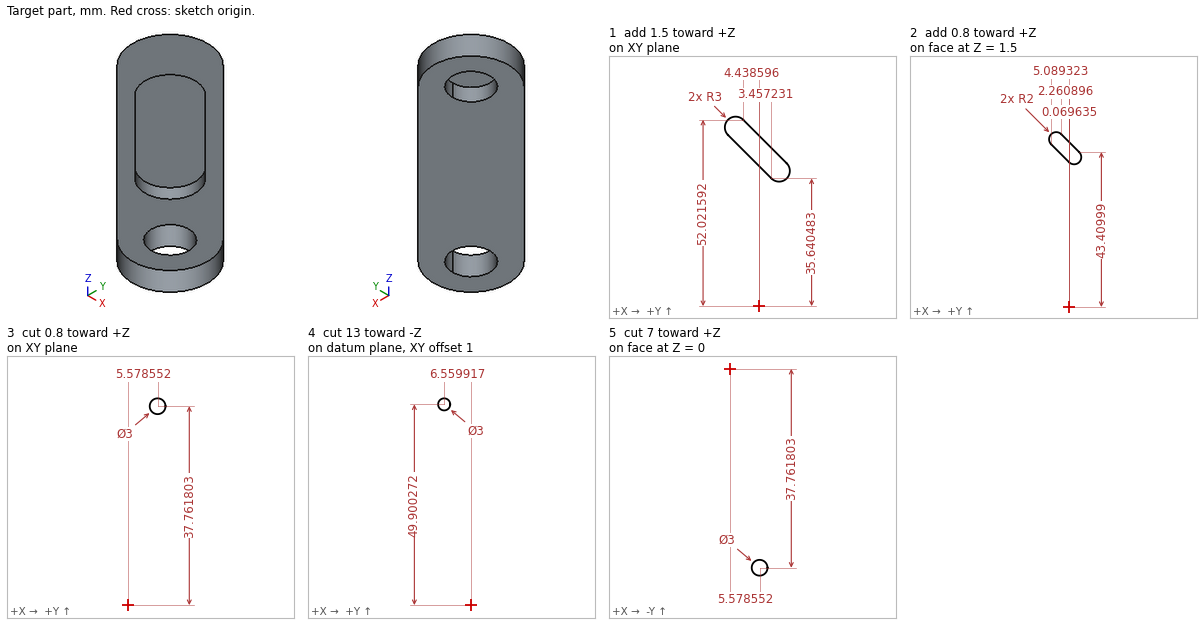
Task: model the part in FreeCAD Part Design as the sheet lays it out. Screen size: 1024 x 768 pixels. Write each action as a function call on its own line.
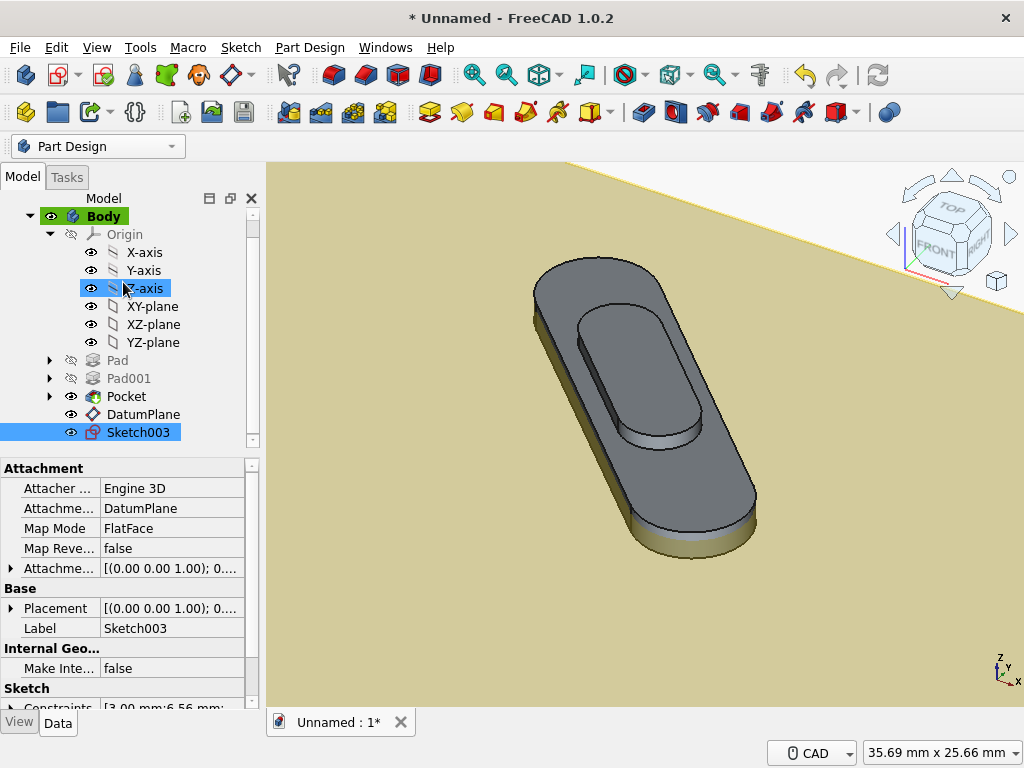
click(644, 112)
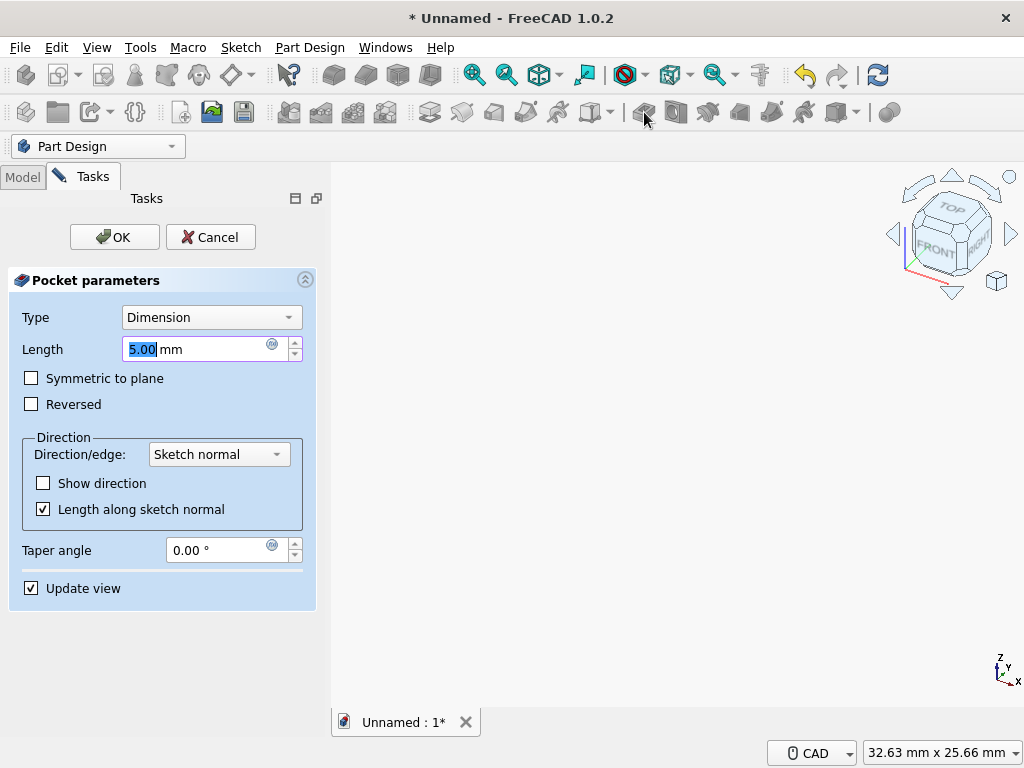
text(13)
key(Tab)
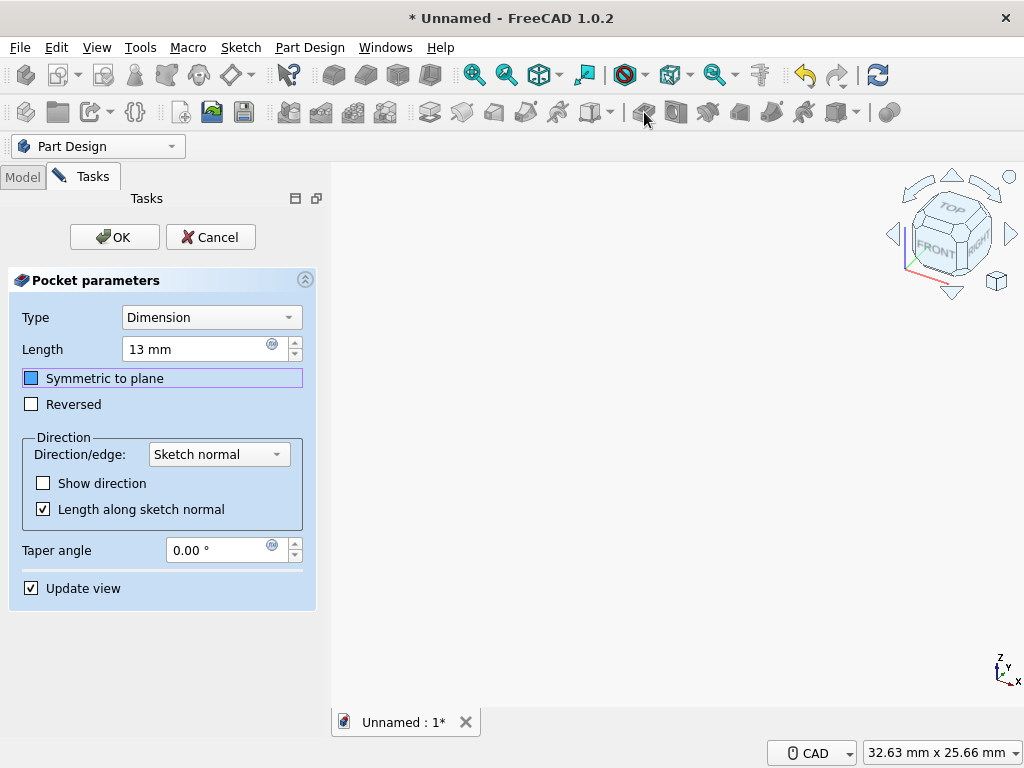
click(115, 237)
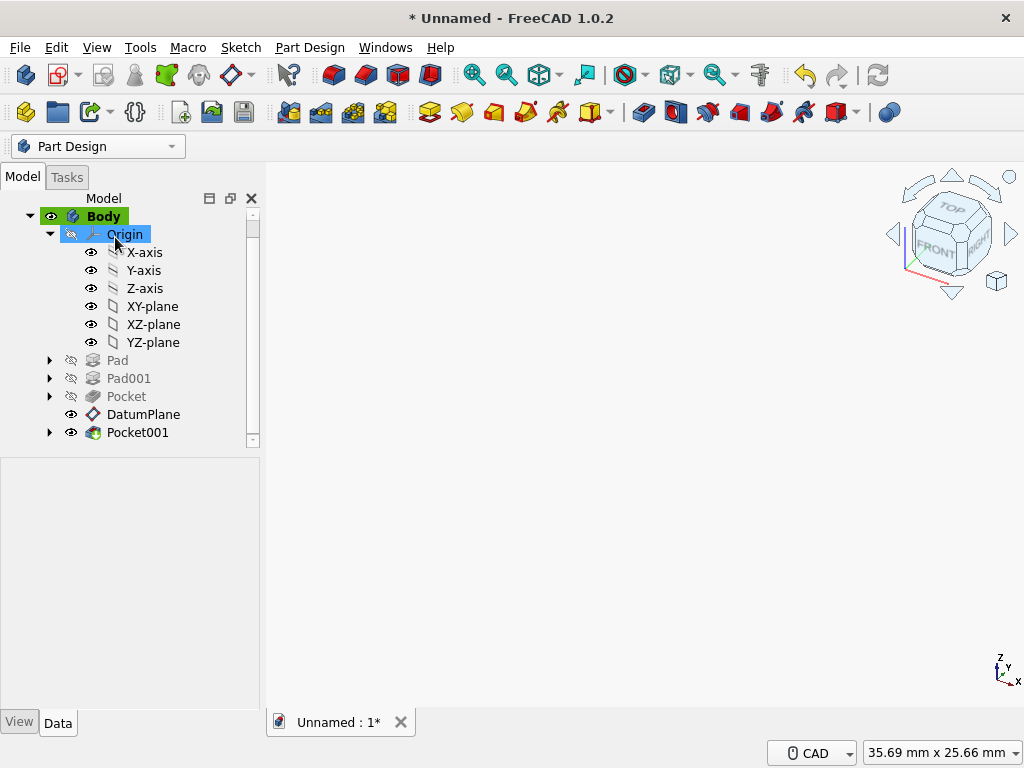
click(116, 414)
key(space)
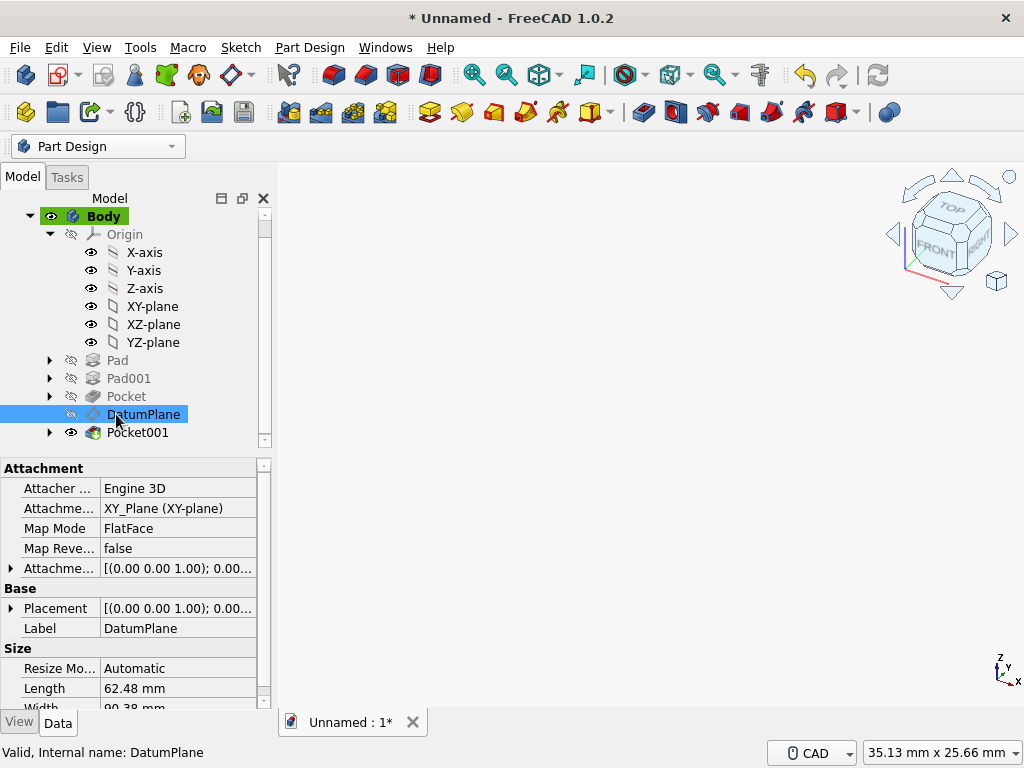
key(v)
key(f)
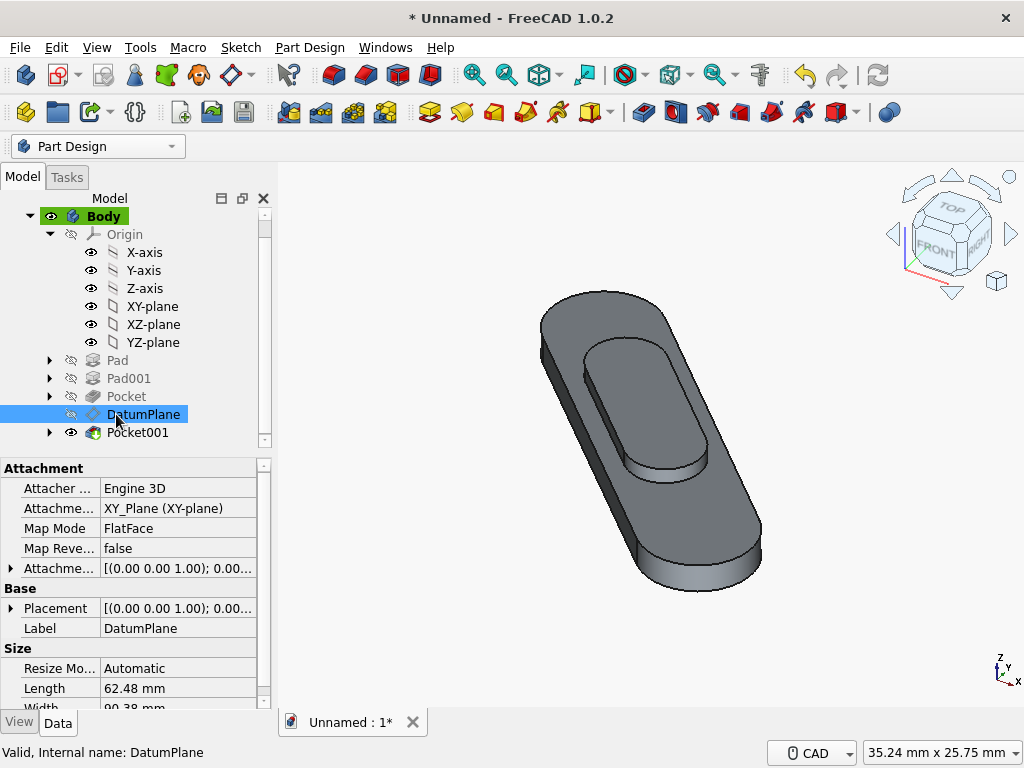
key(5)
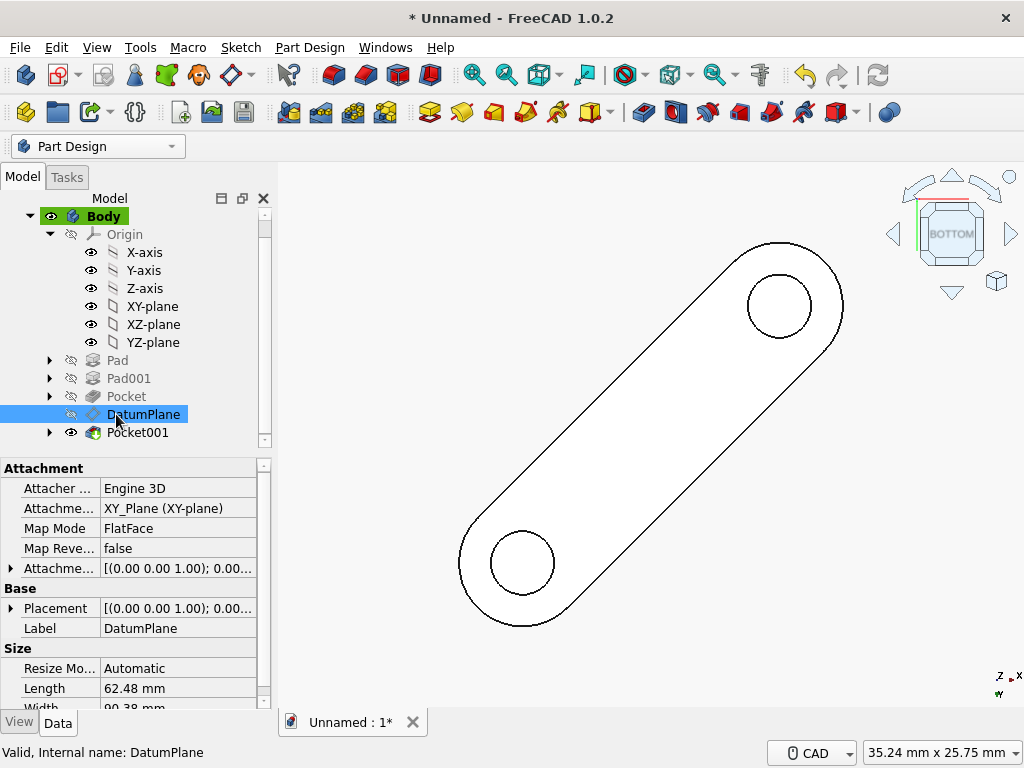
click(651, 433)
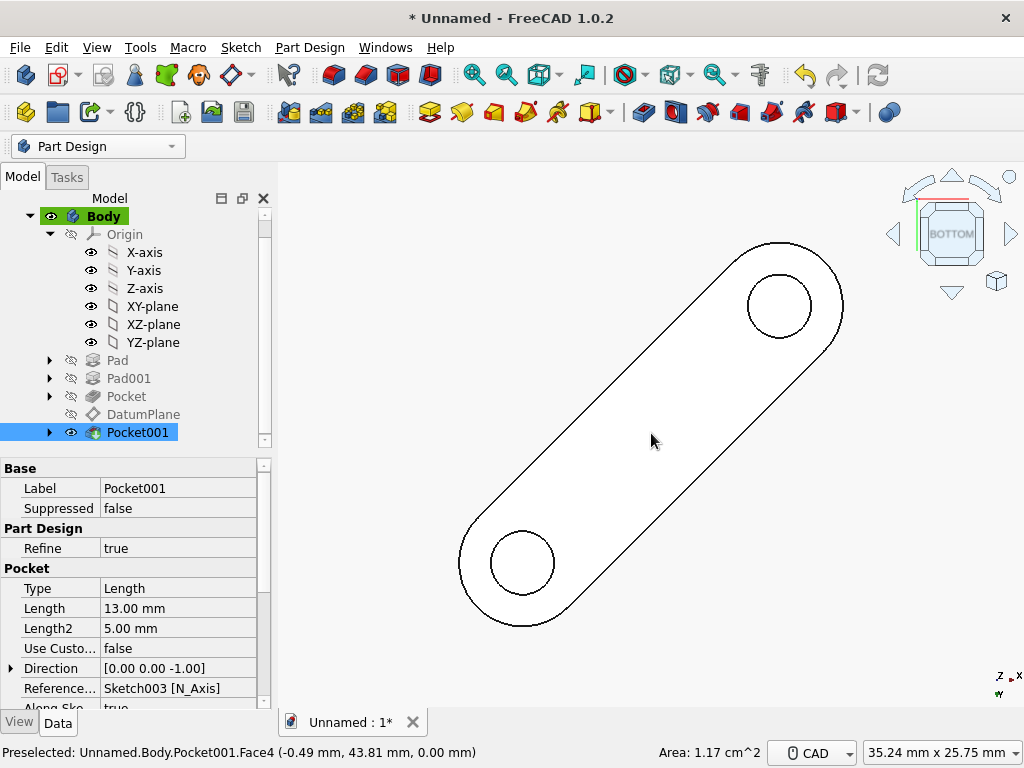
click(58, 76)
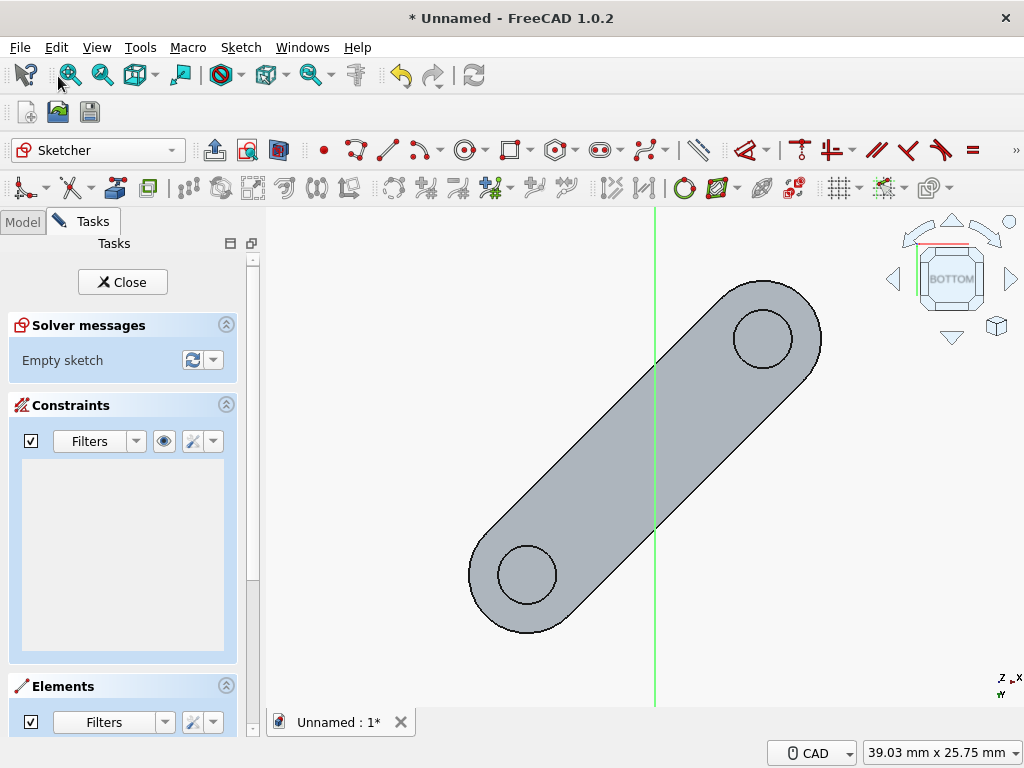
scroll(810, 309, up, 8)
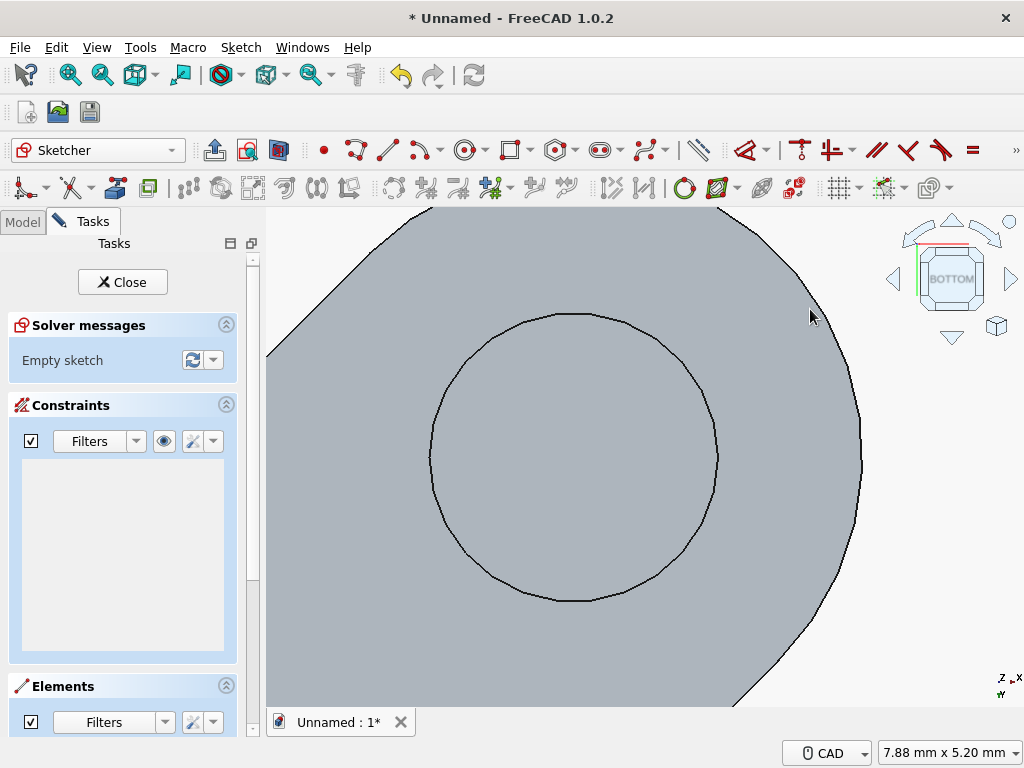
click(466, 150)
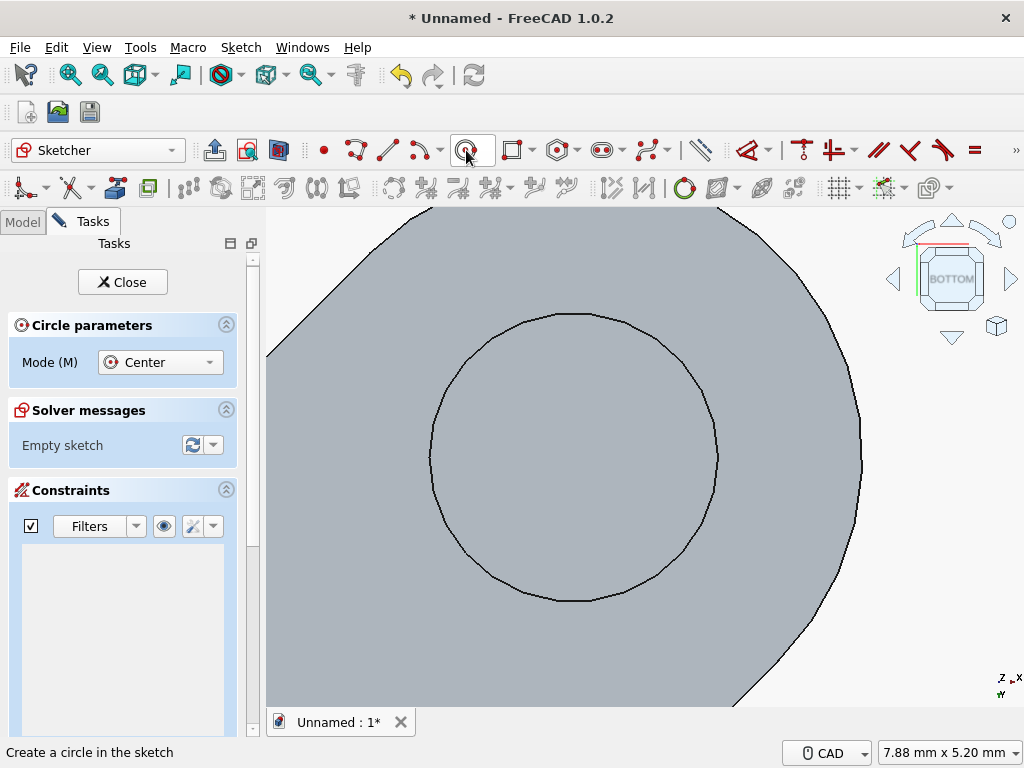
click(574, 457)
click(676, 355)
key(Escape)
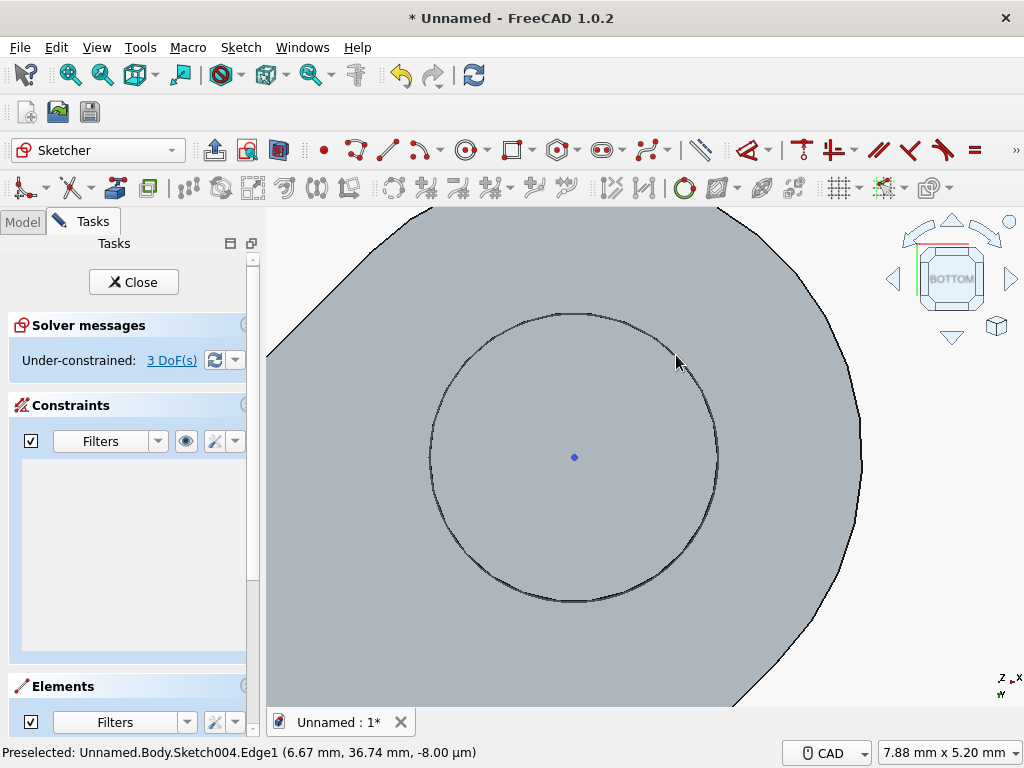
click(748, 150)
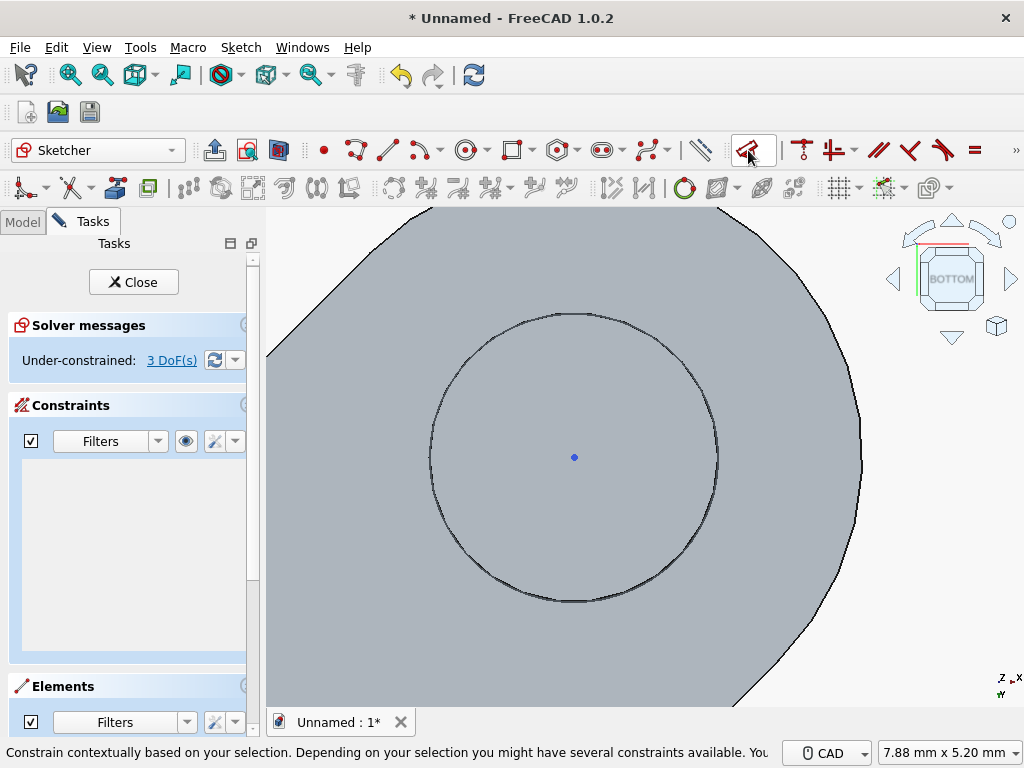
click(676, 356)
click(699, 333)